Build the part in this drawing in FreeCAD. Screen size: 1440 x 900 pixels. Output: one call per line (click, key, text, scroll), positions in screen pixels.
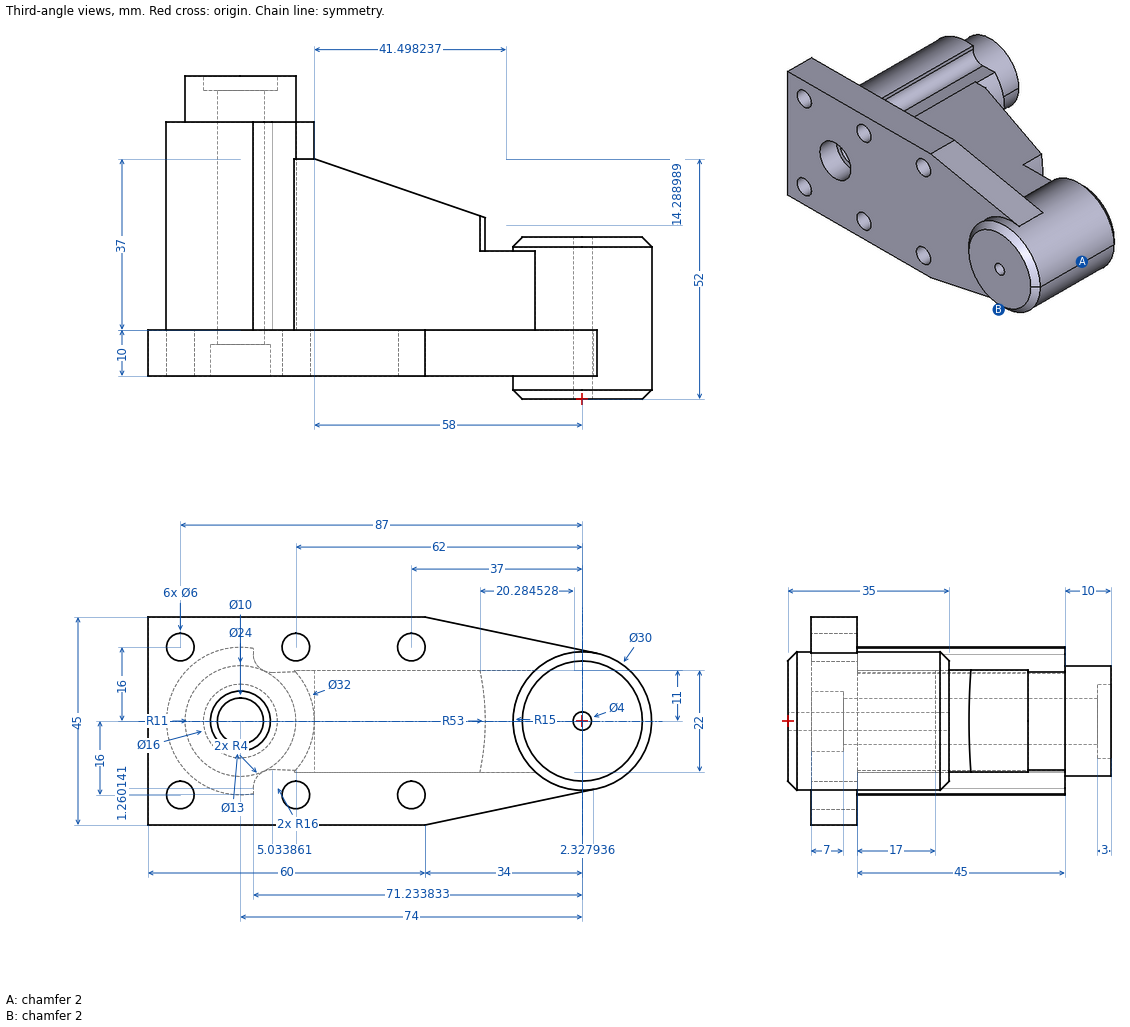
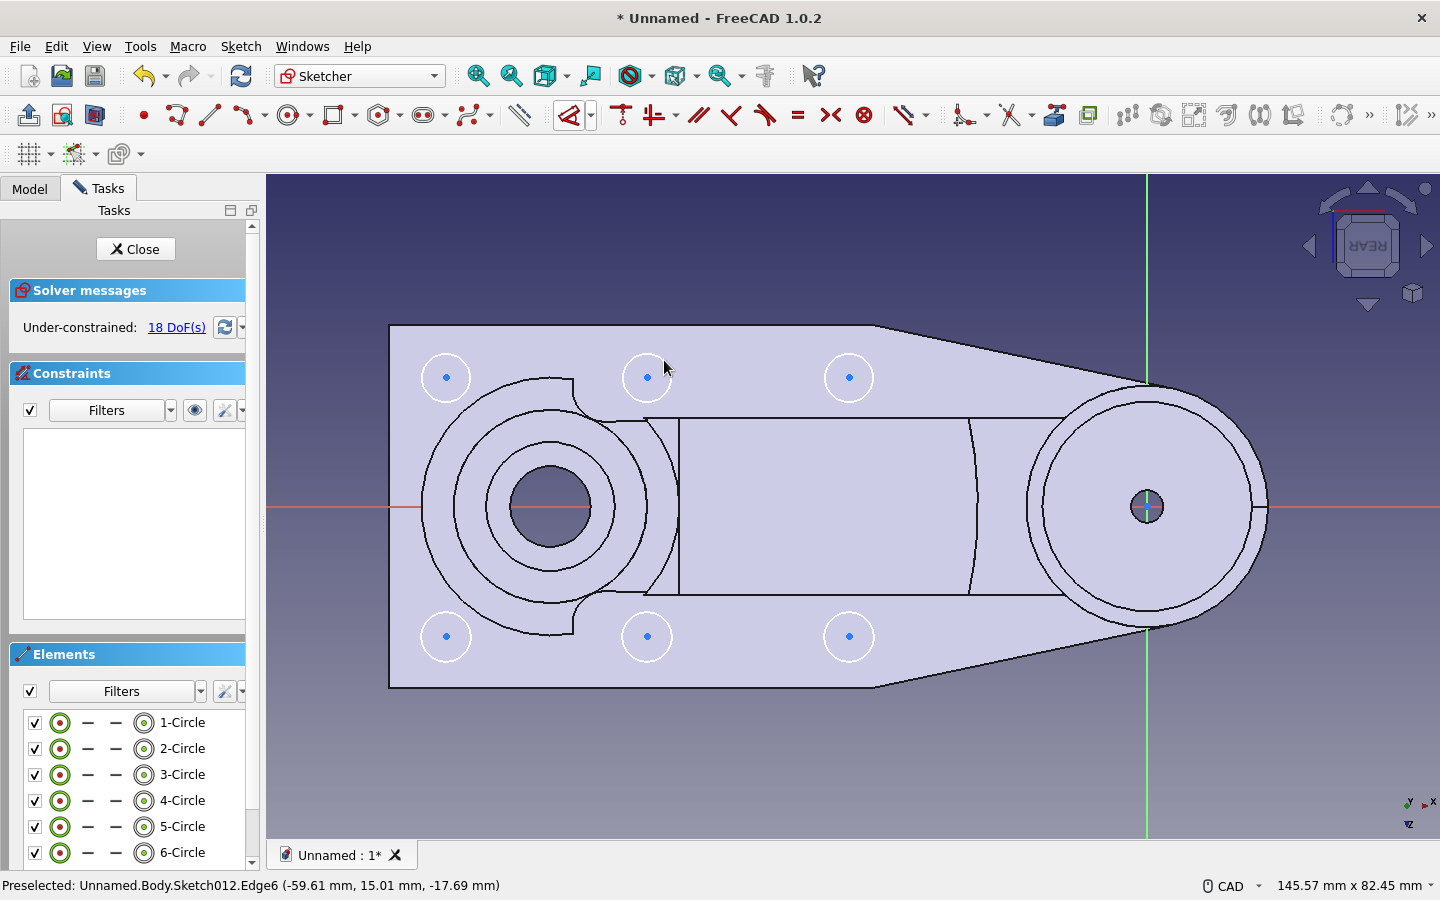
click(463, 619)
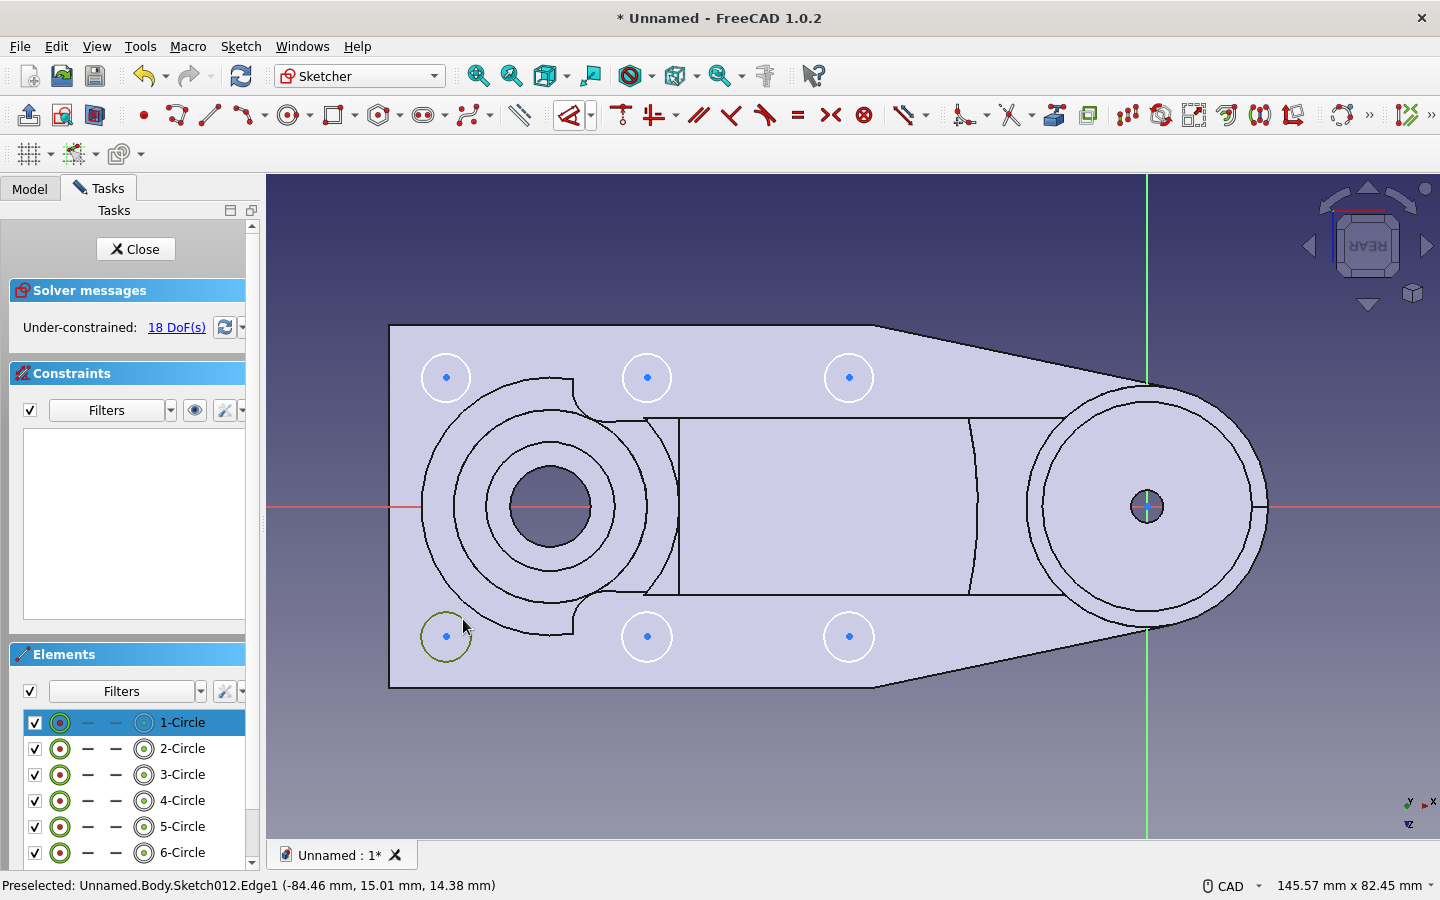
click(664, 619)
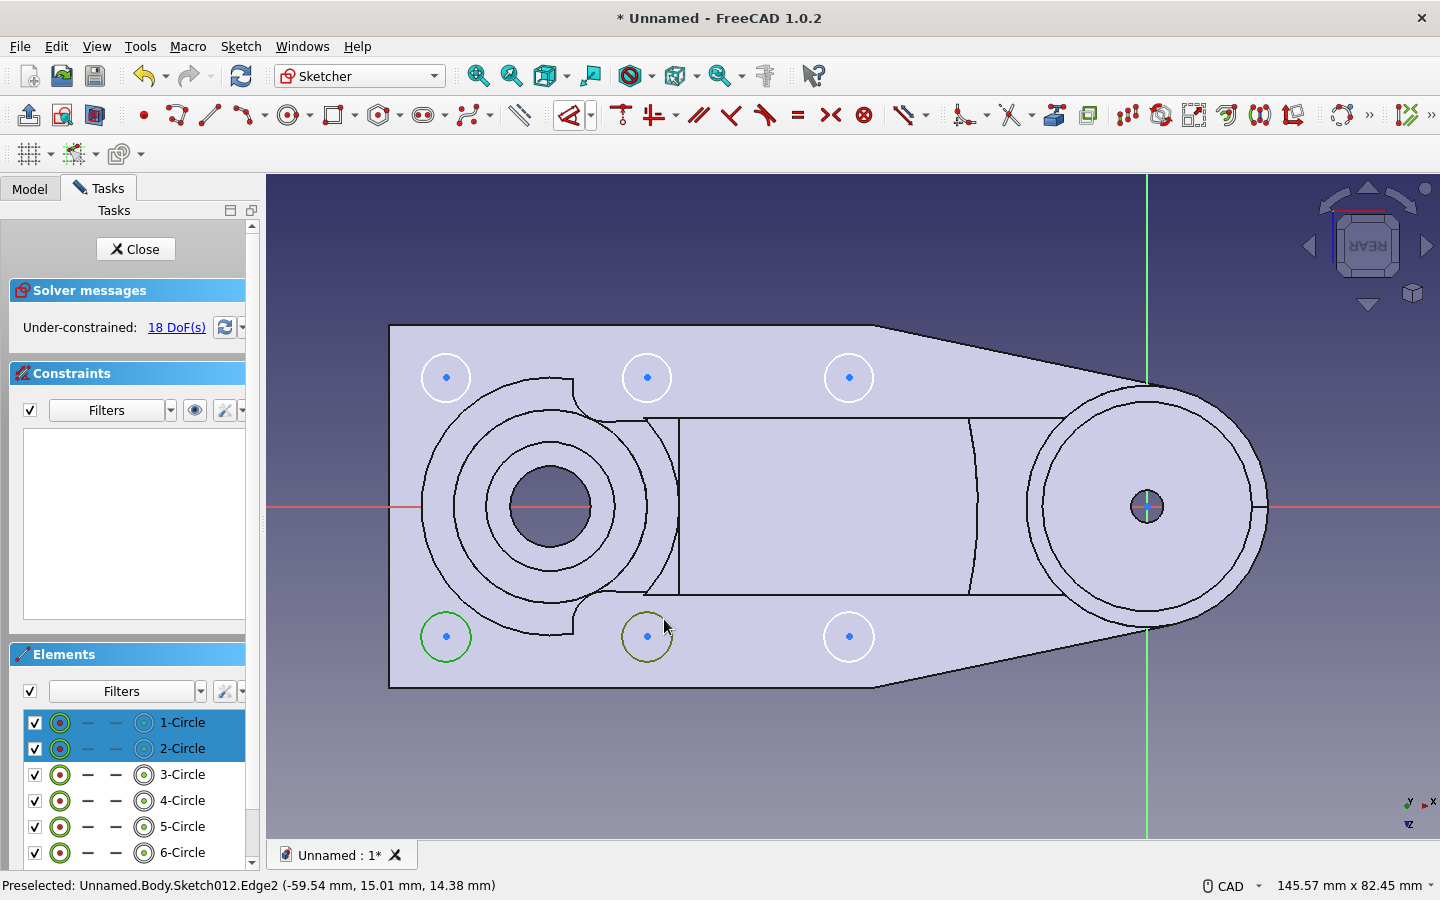
click(866, 619)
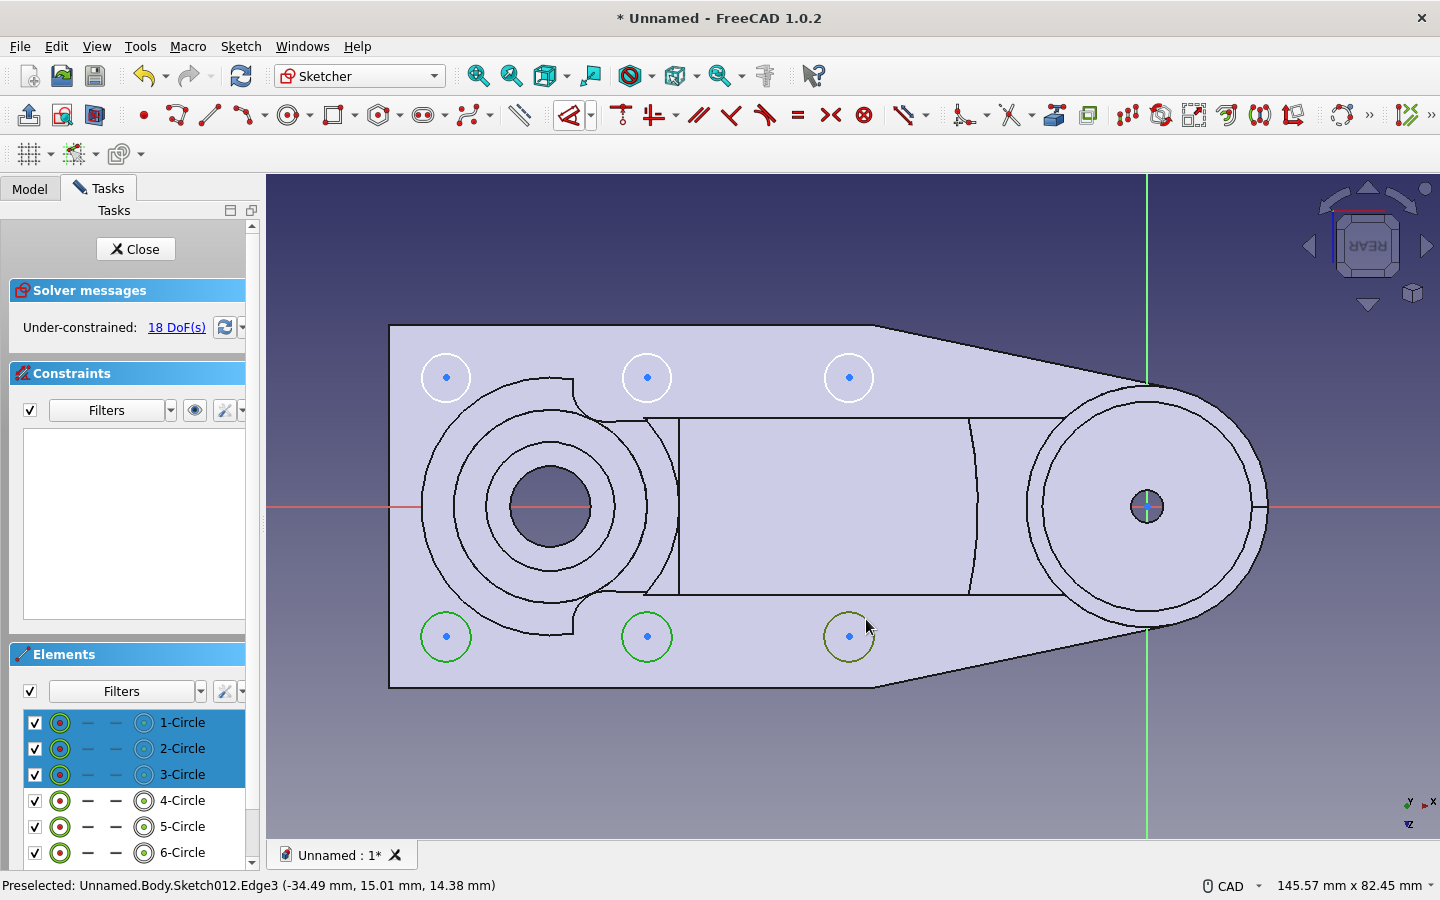
click(463, 361)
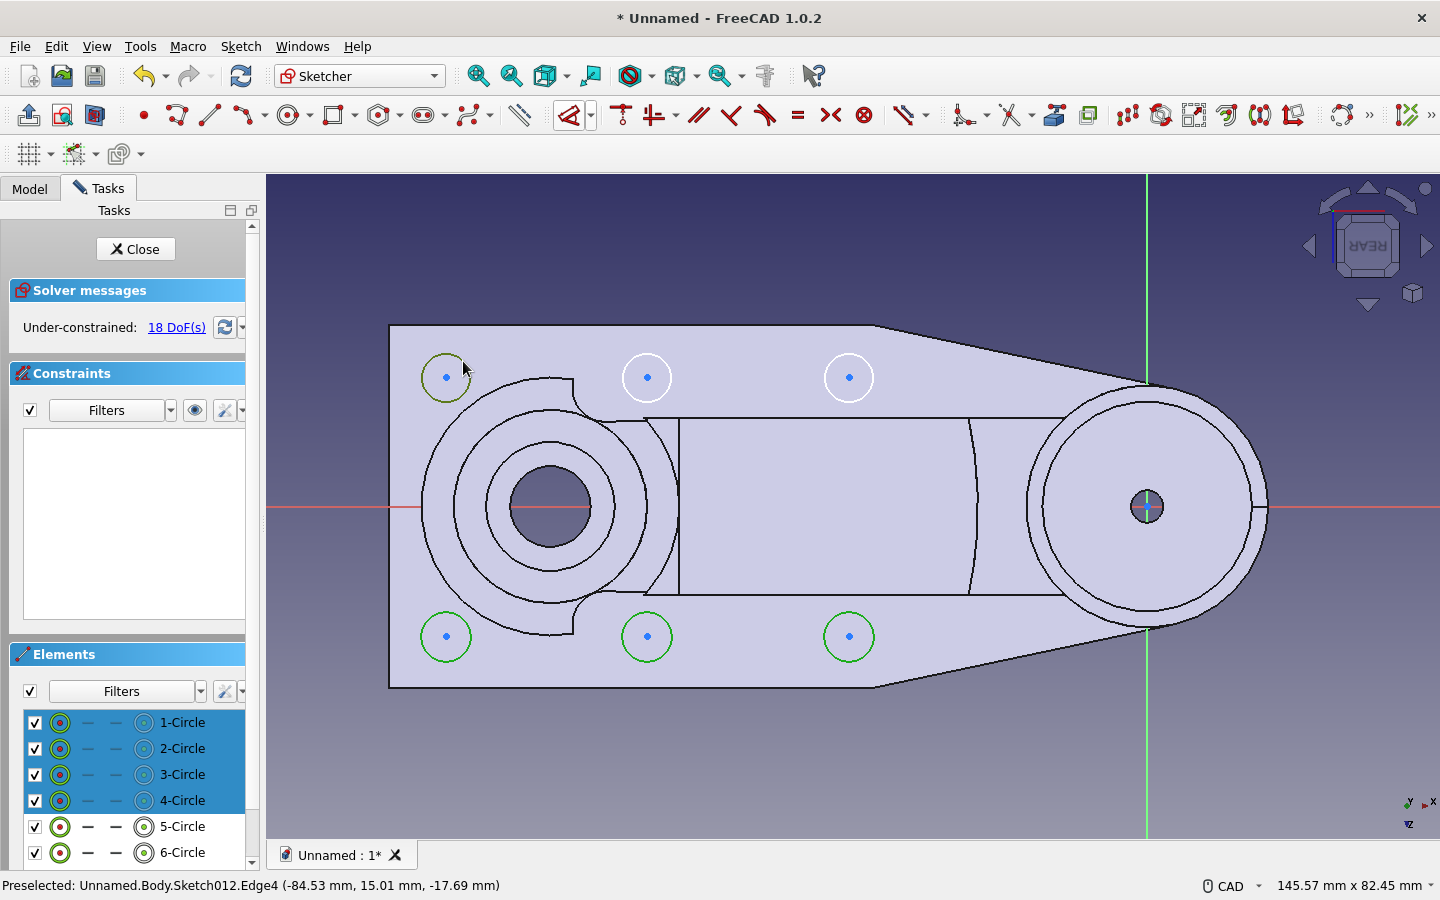
click(866, 361)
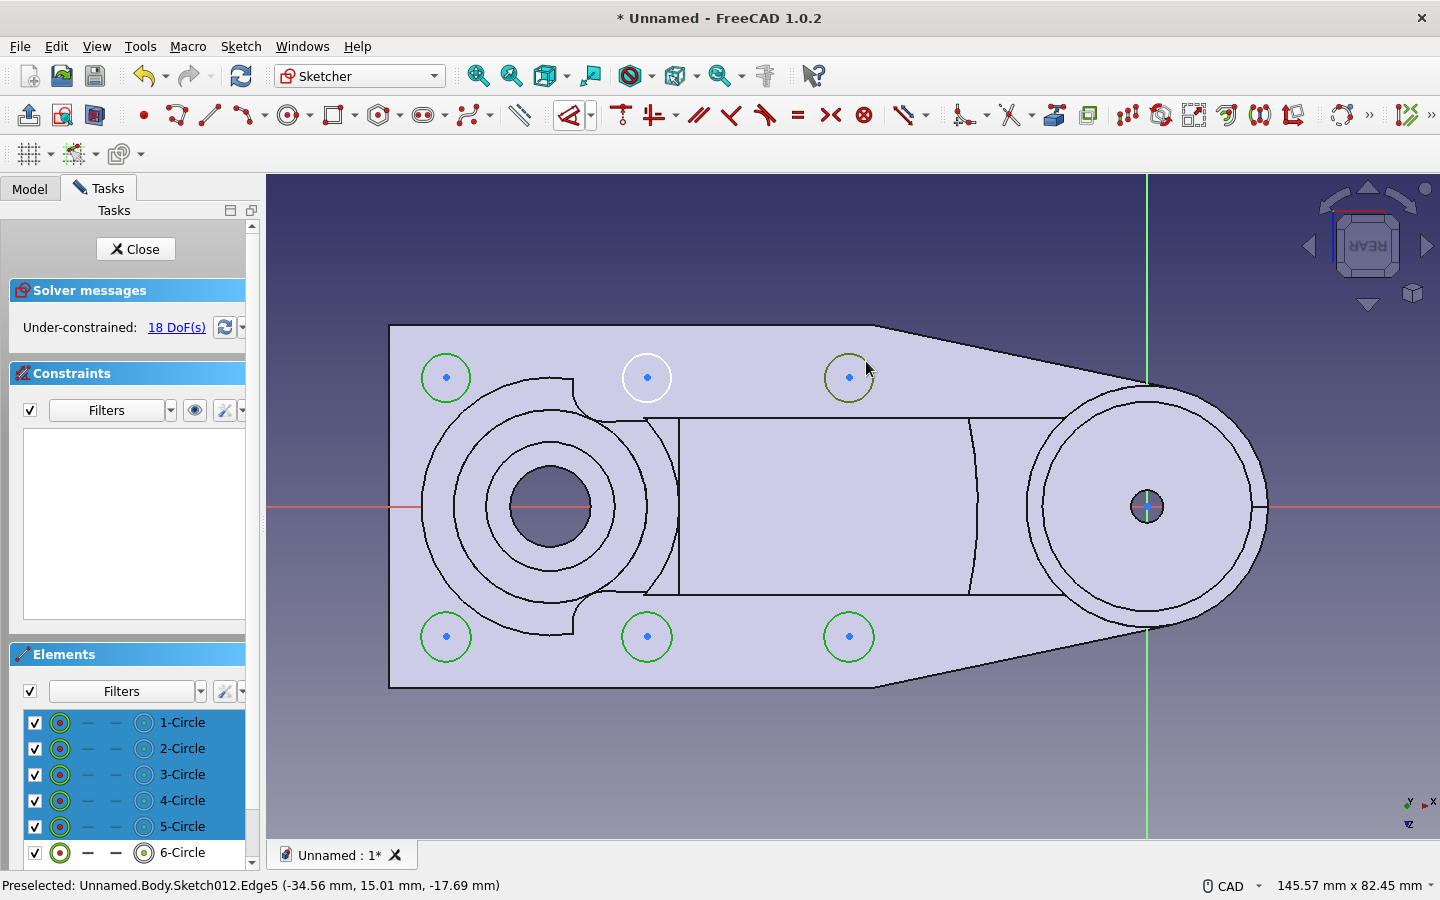
click(664, 361)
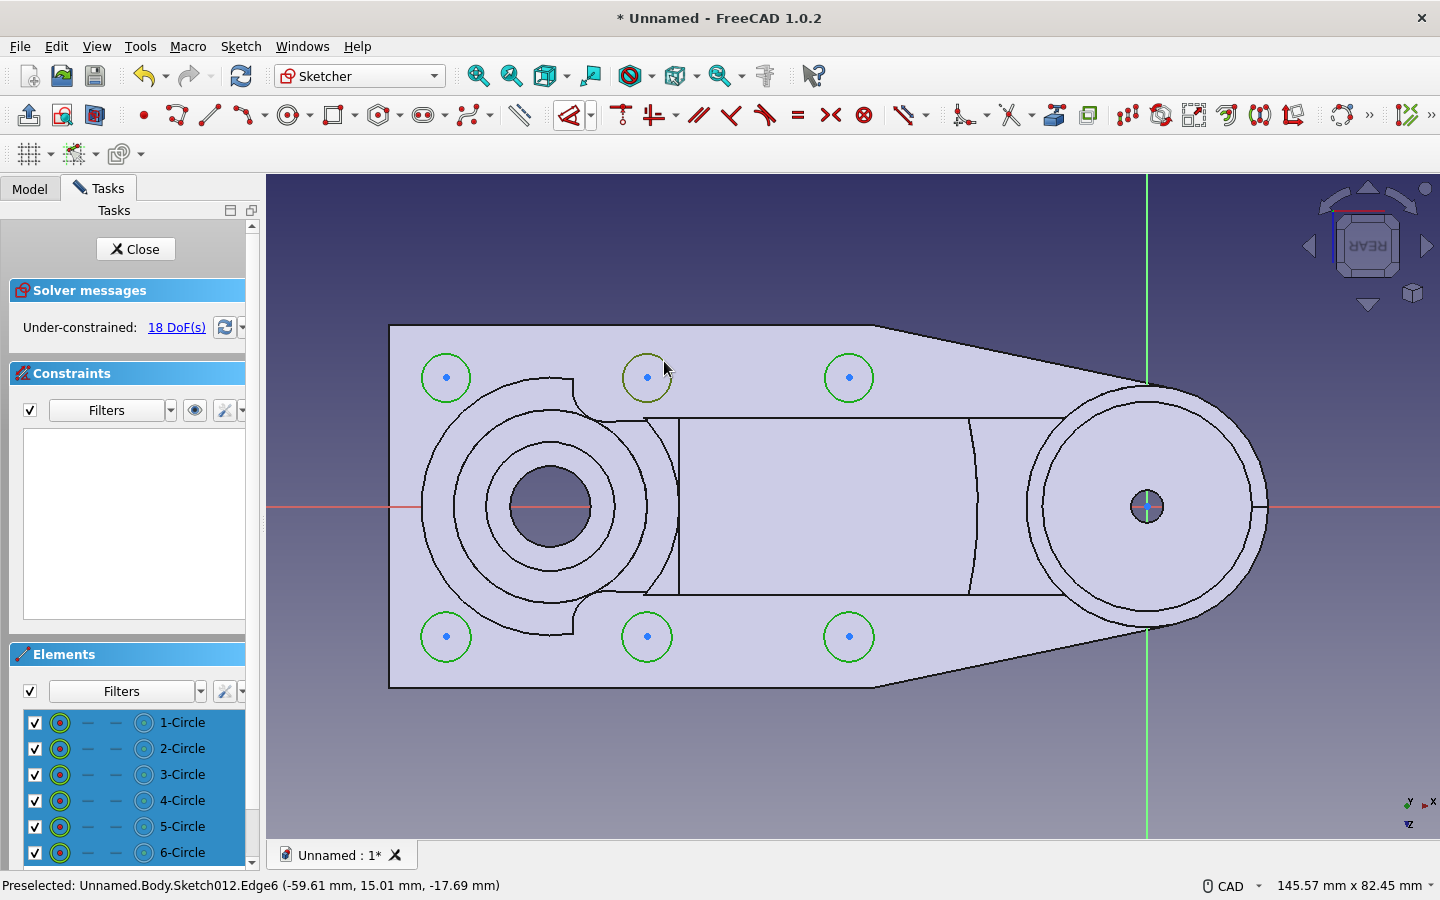
click(798, 116)